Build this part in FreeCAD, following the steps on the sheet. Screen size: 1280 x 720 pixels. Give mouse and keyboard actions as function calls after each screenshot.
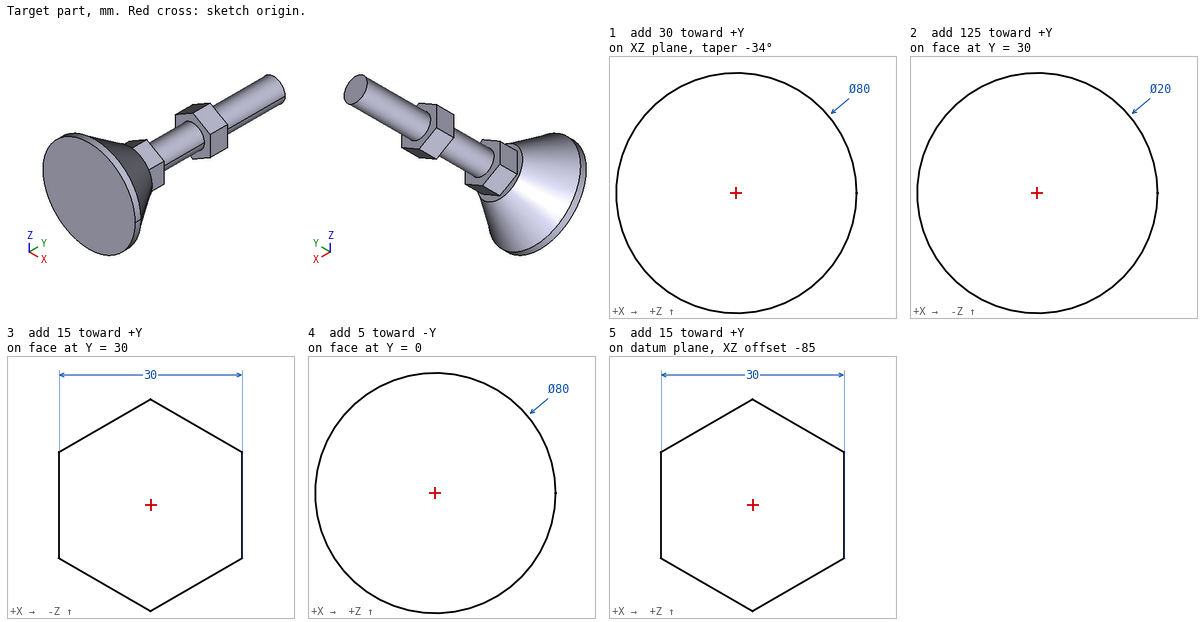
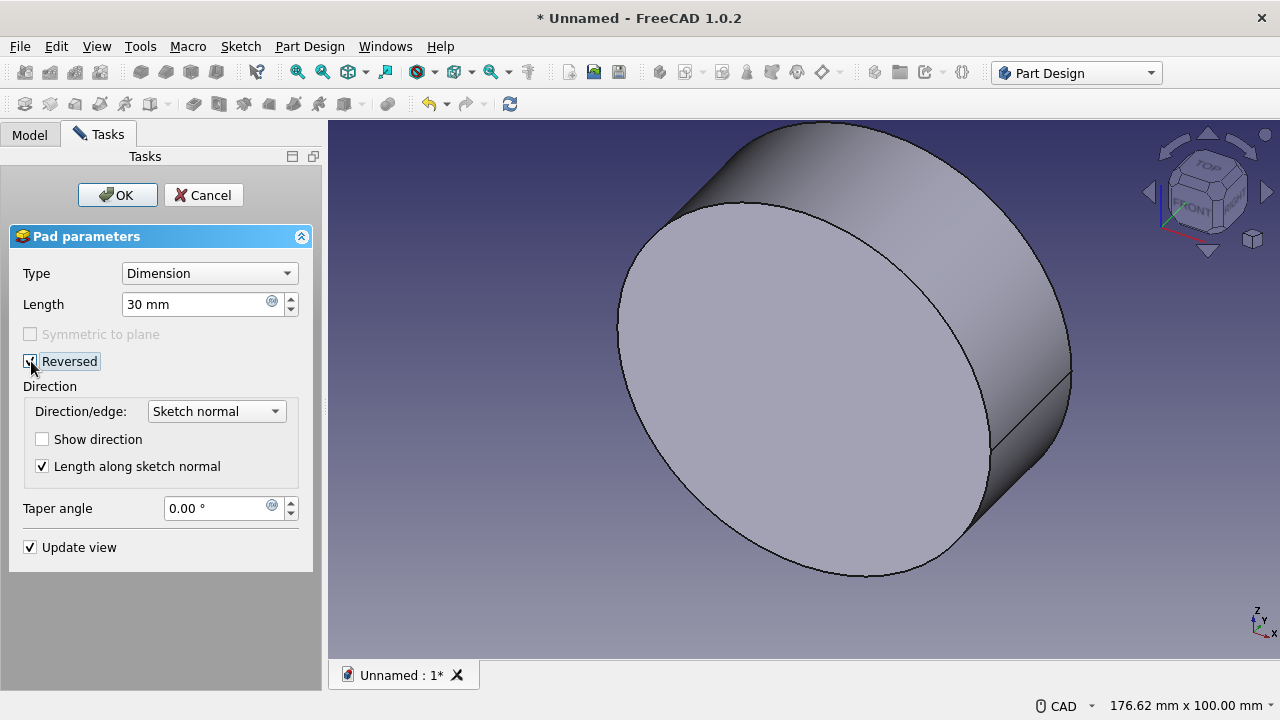
triple_click(224, 508)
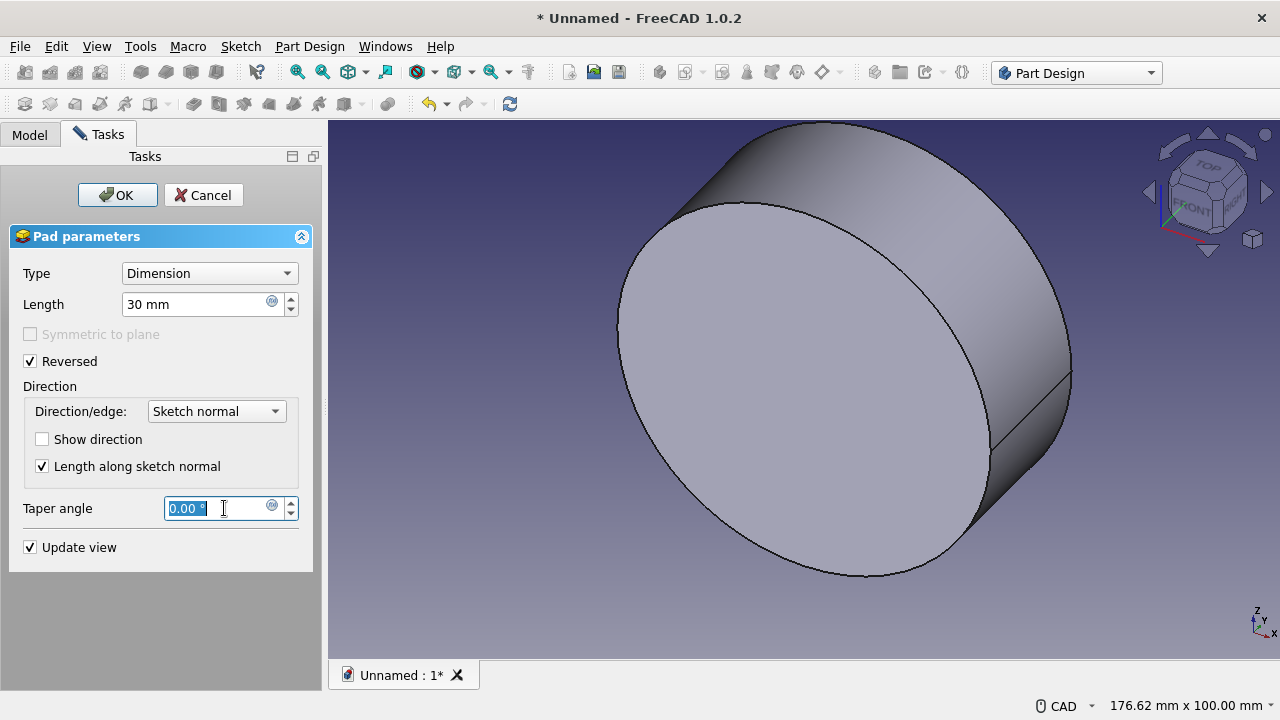
text(-34)
key(Tab)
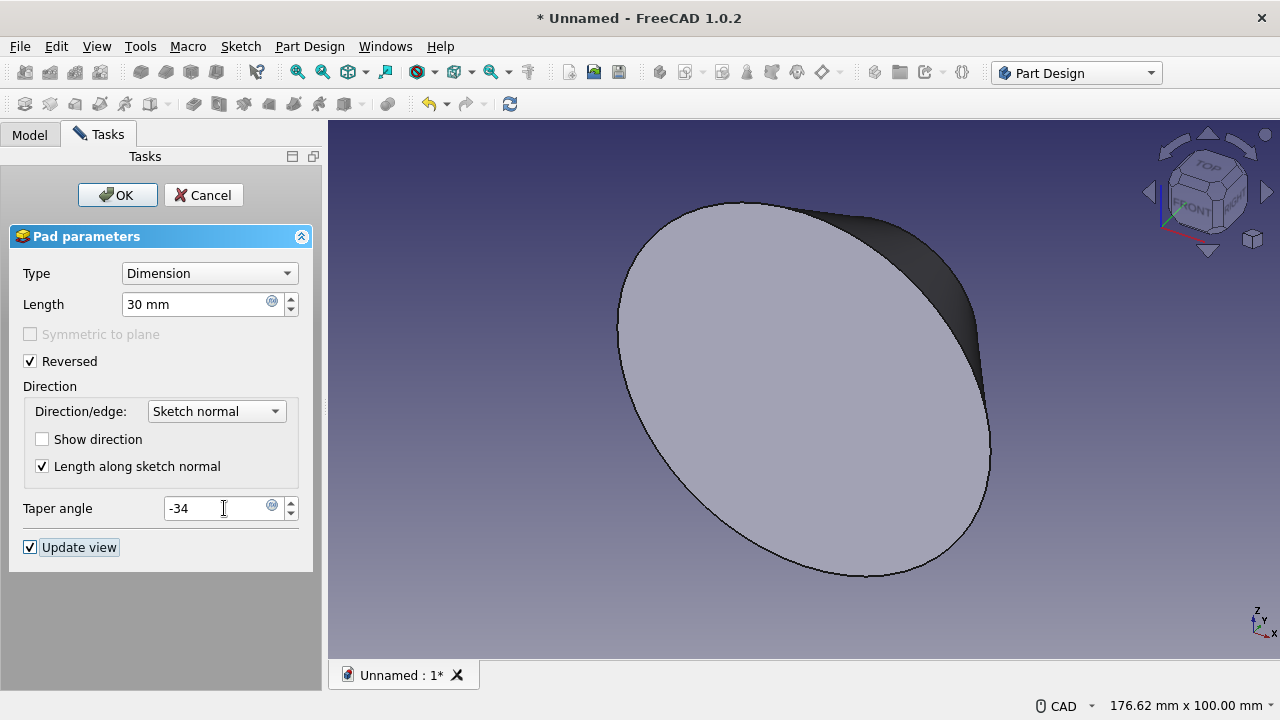
click(118, 195)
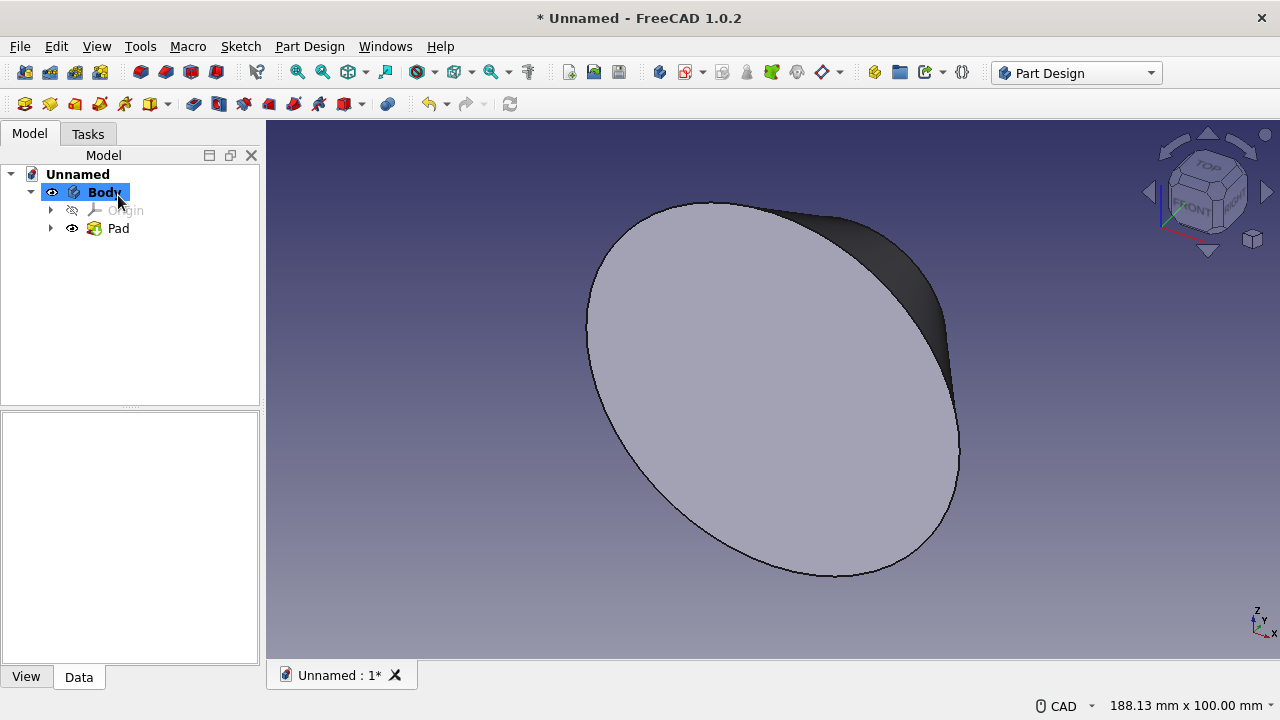
click(298, 72)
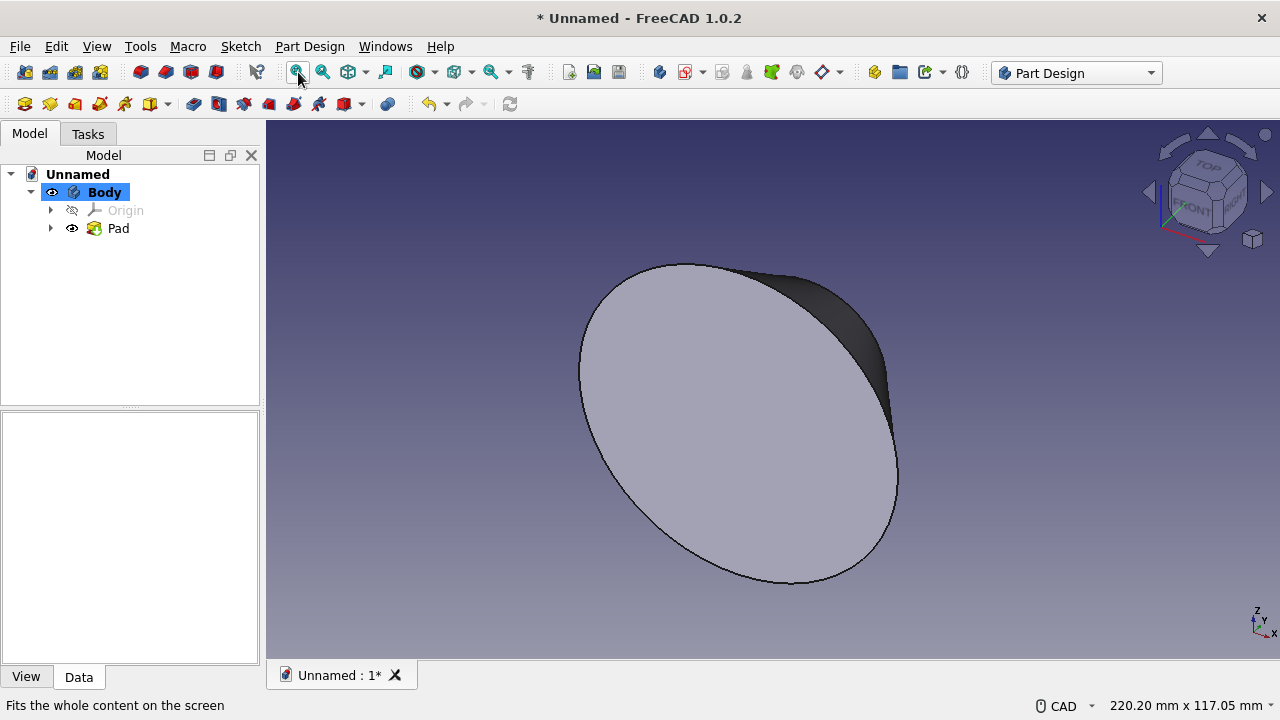
key(4)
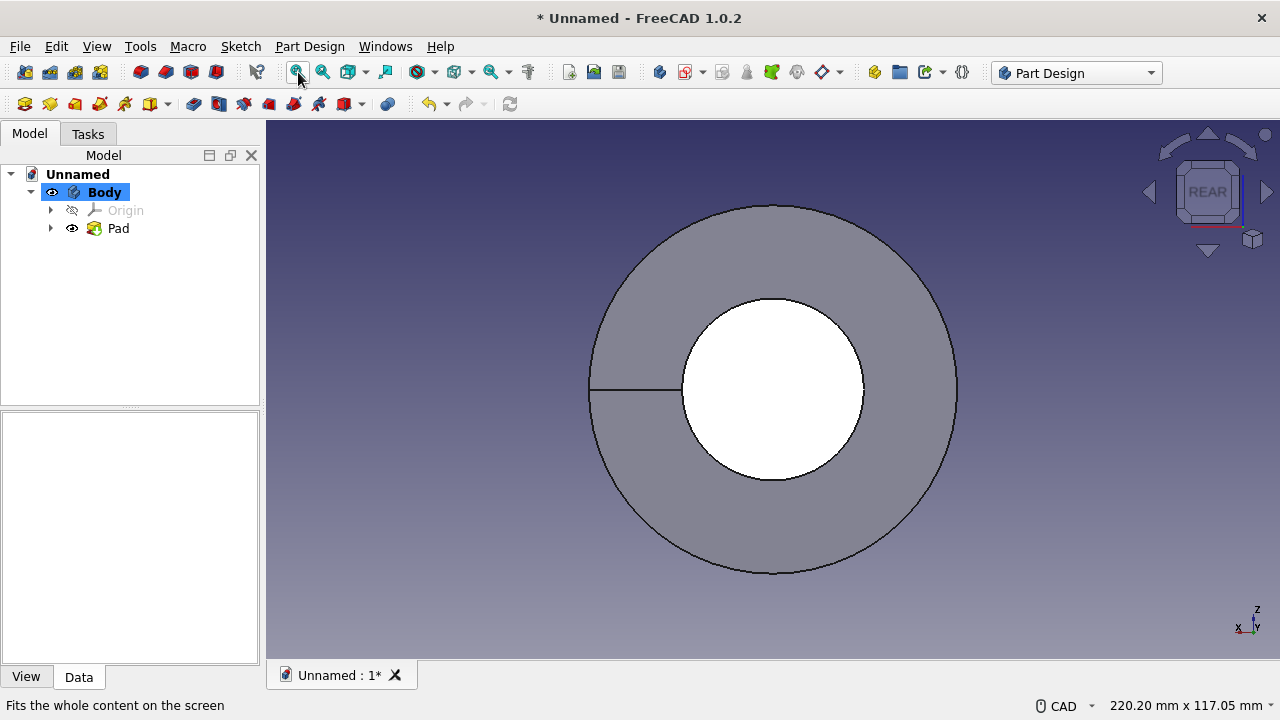
click(773, 389)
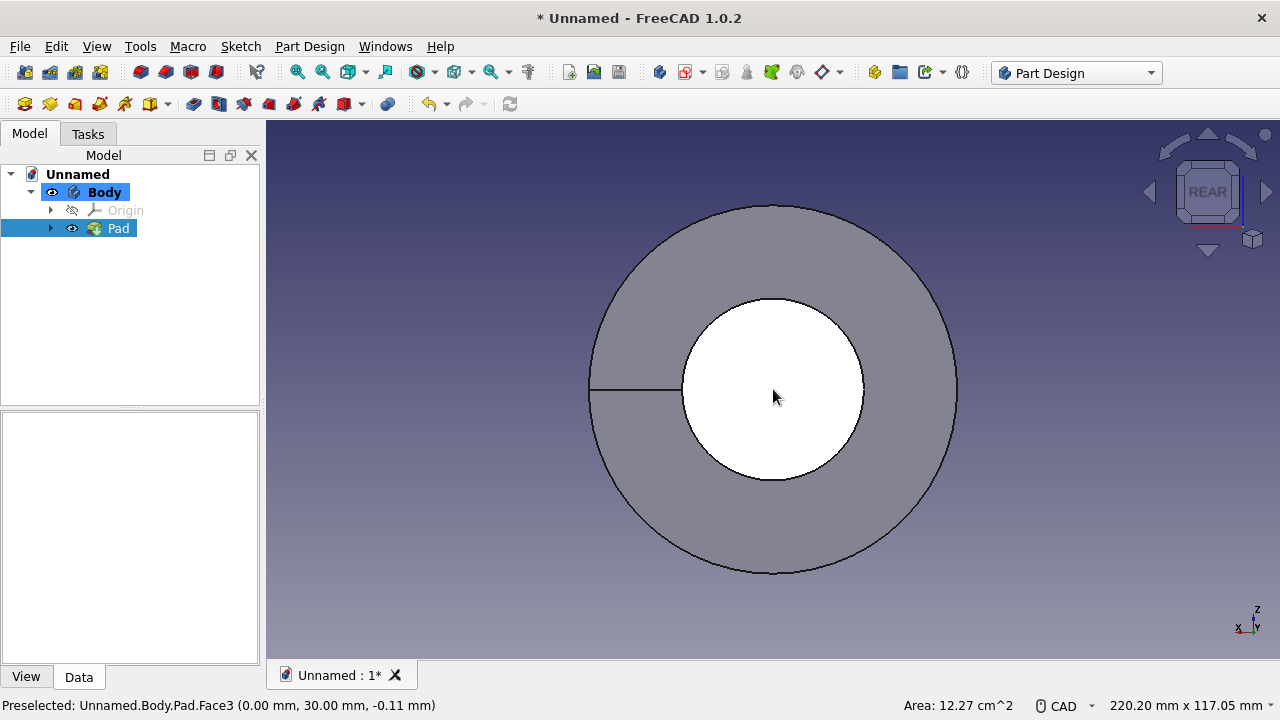
click(684, 72)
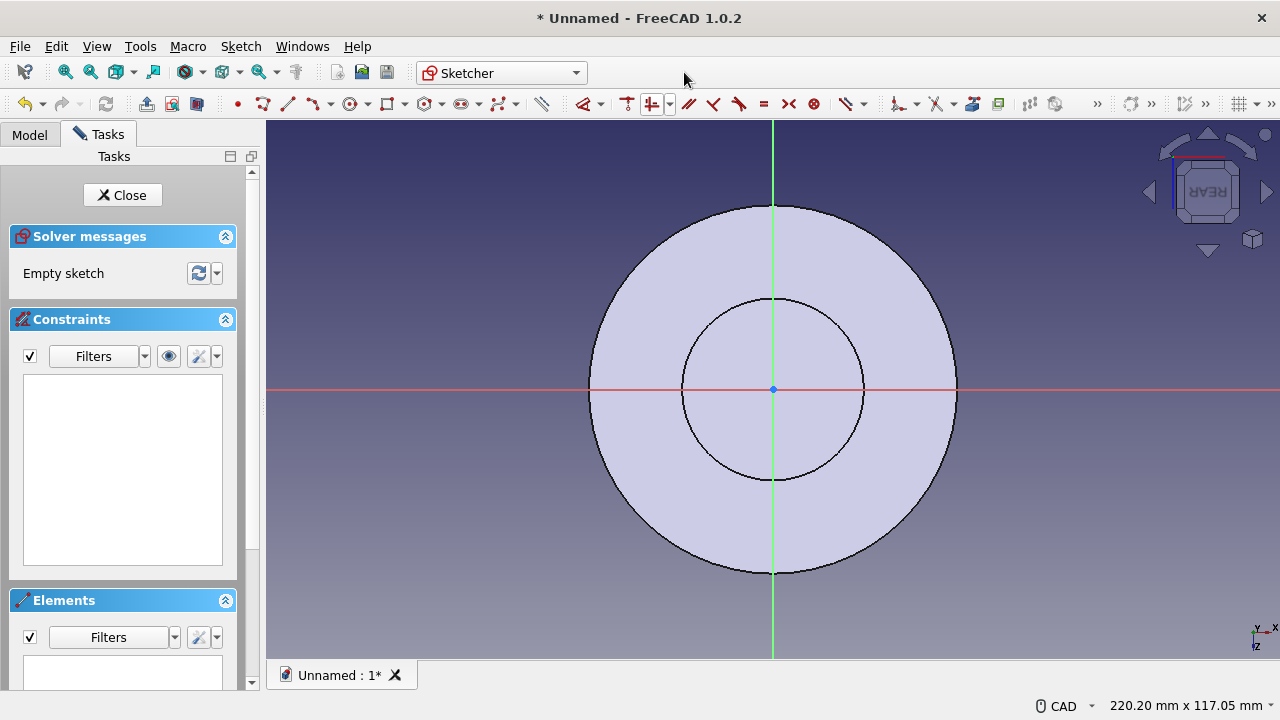
scroll(795, 389, up, 7)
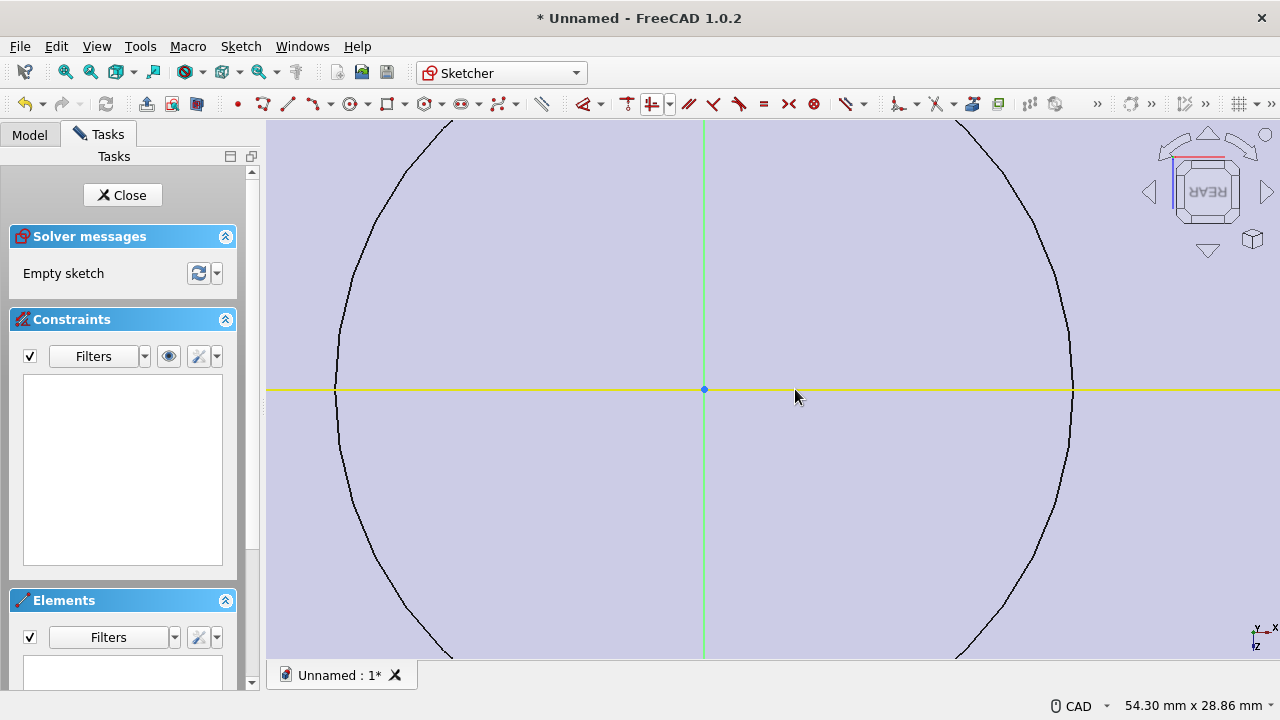
click(350, 104)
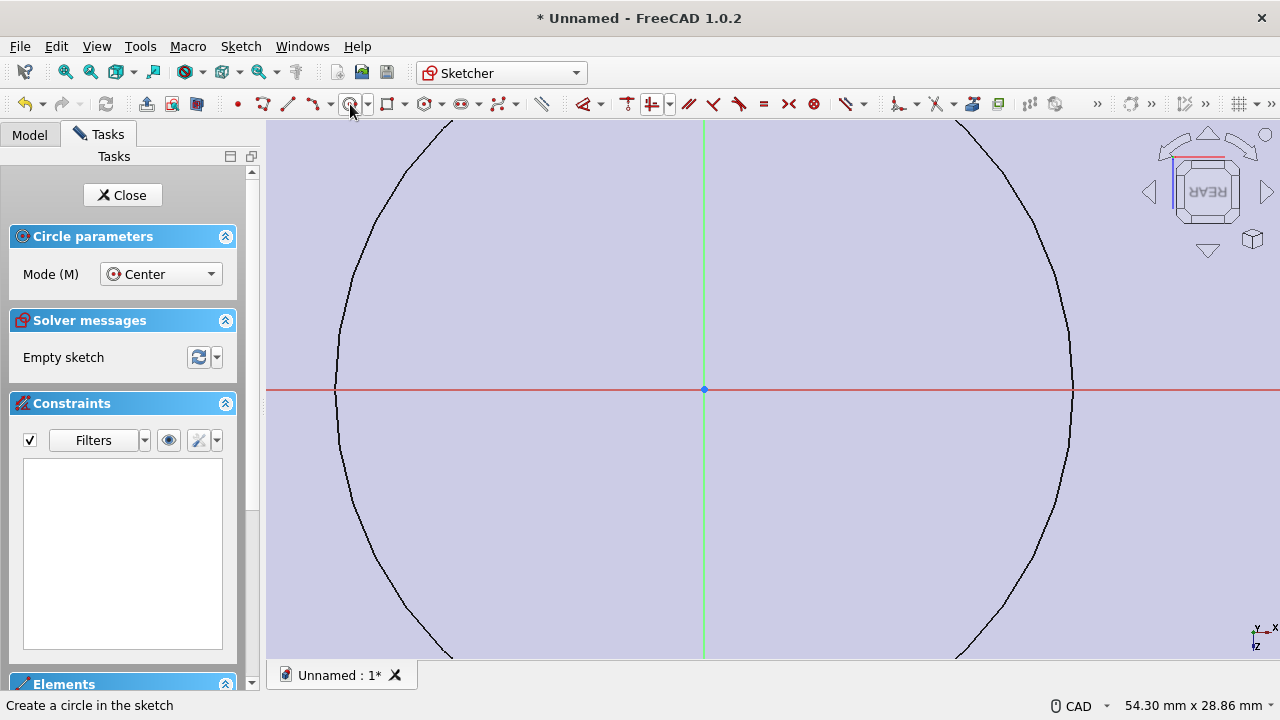
click(704, 389)
move(836, 257)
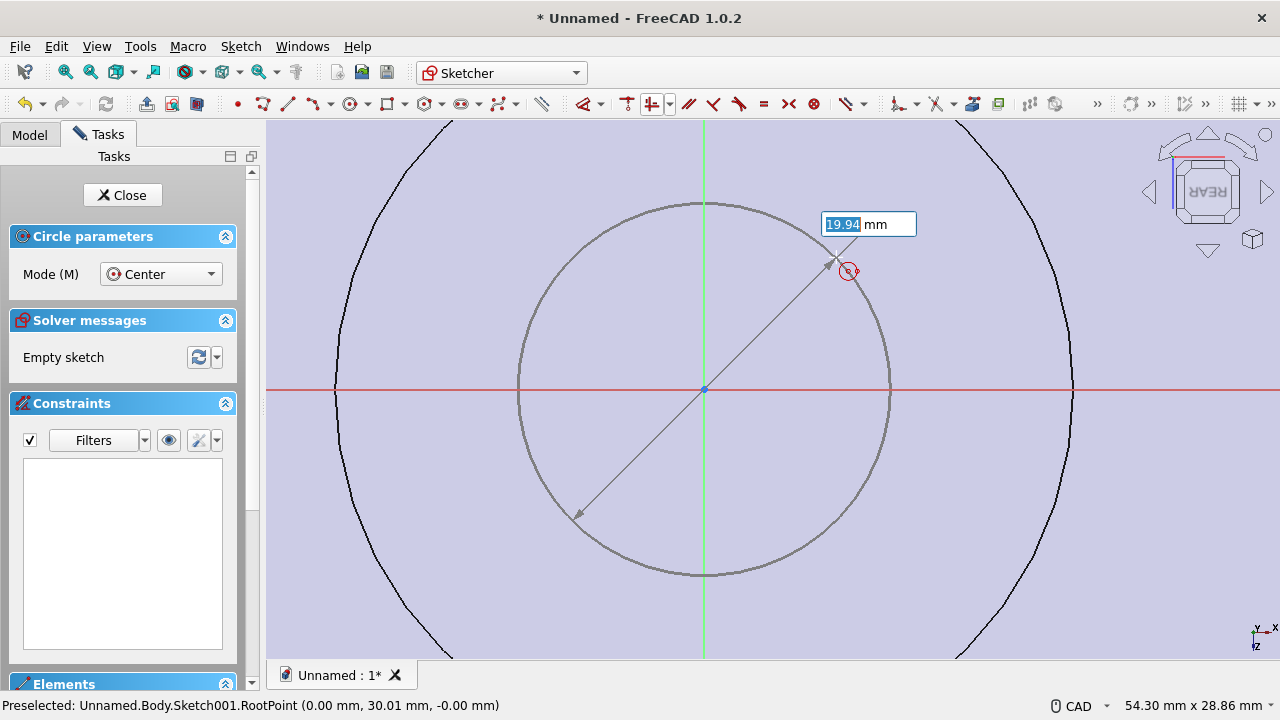
text(20)
key(Return)
key(Escape)